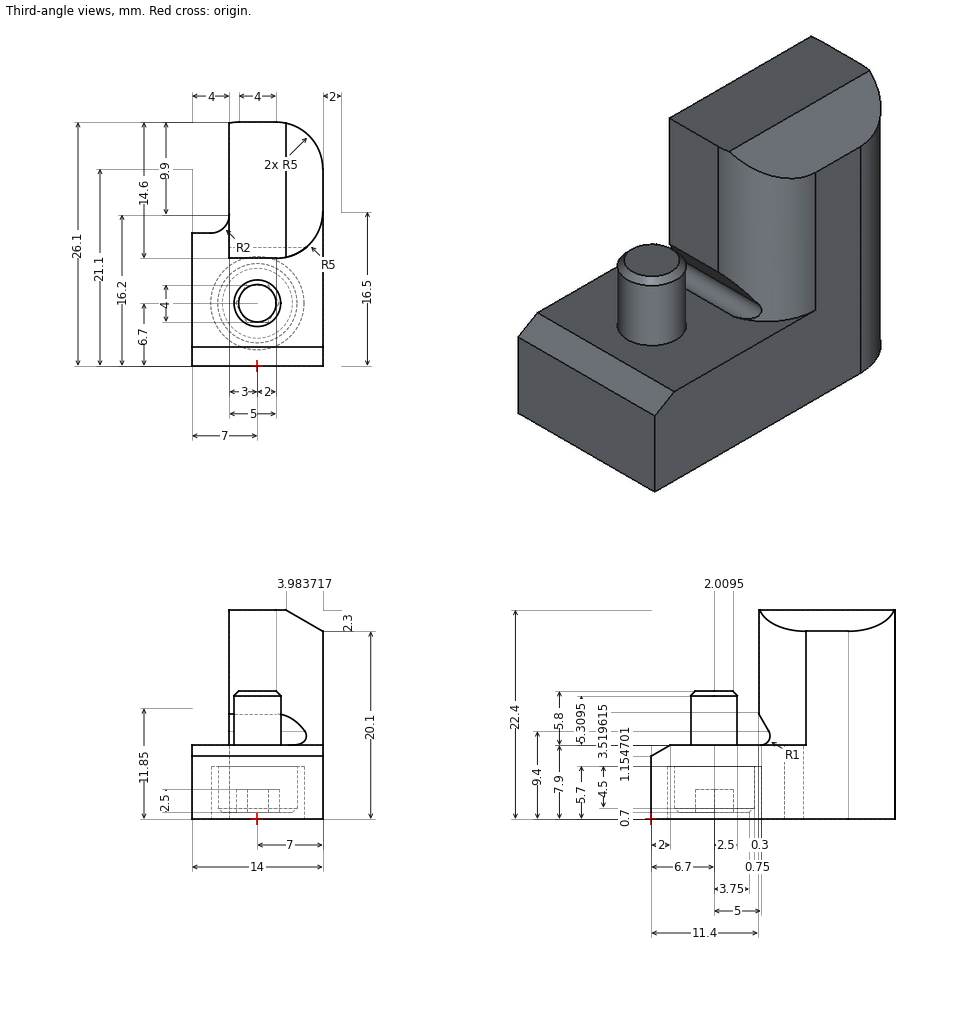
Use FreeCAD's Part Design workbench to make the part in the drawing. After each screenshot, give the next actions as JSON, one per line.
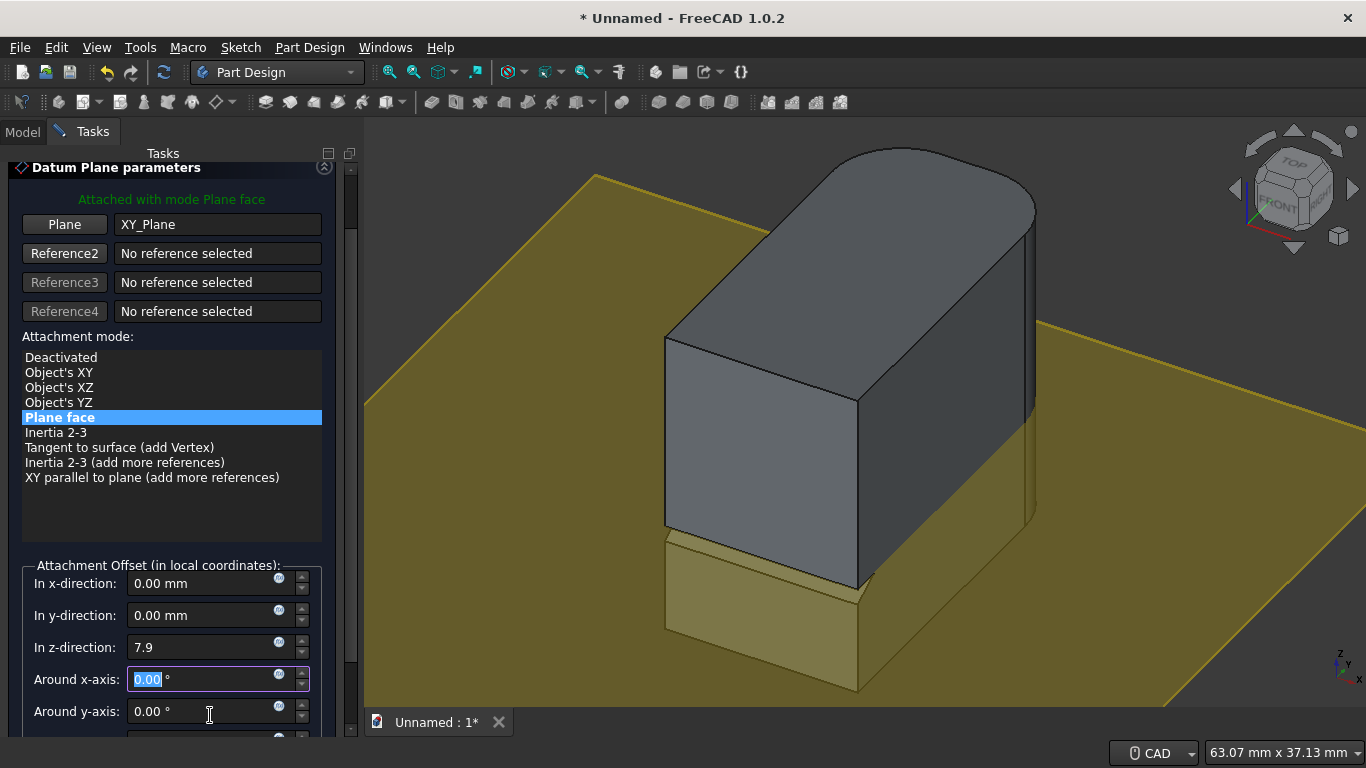
{"action": "scroll", "coordinate": [351, 450], "scroll_direction": "up", "scroll_amount": 2}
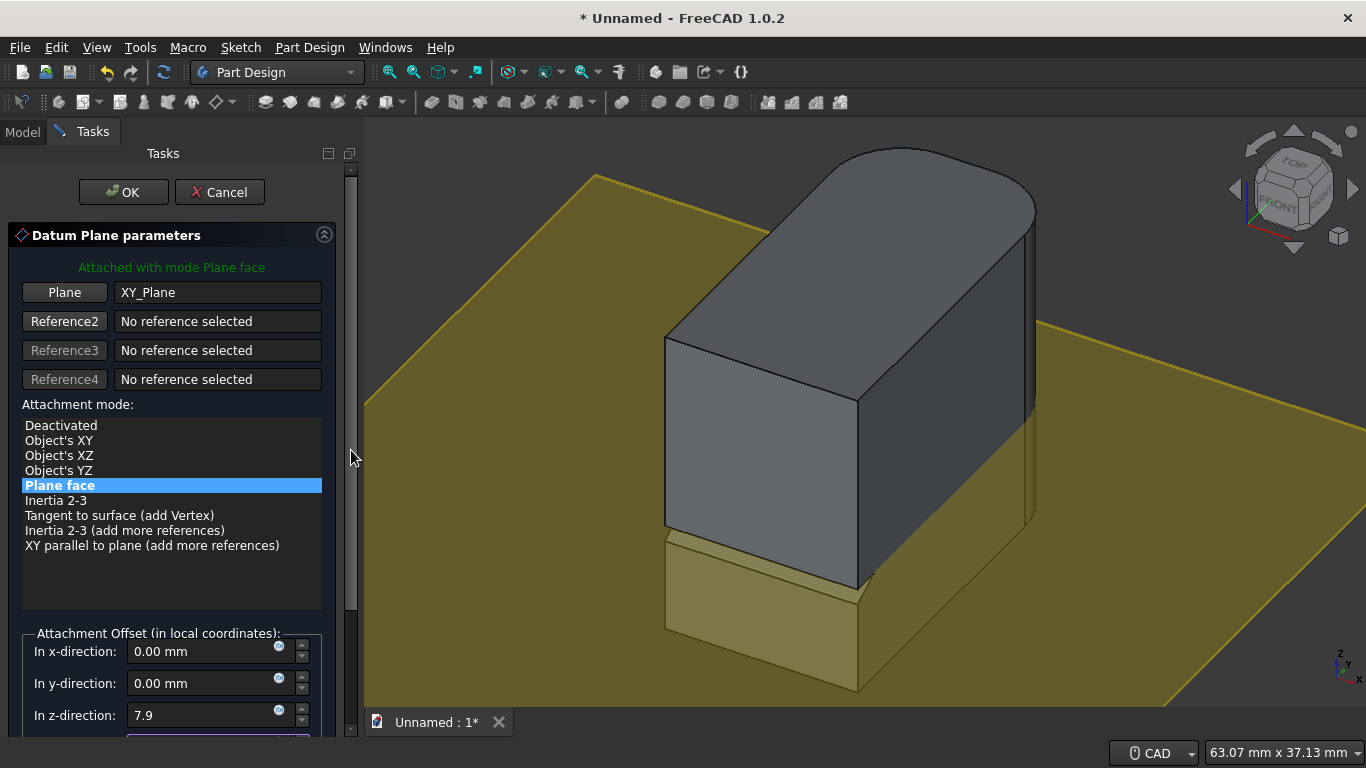
{"action": "left_click", "coordinate": [124, 192]}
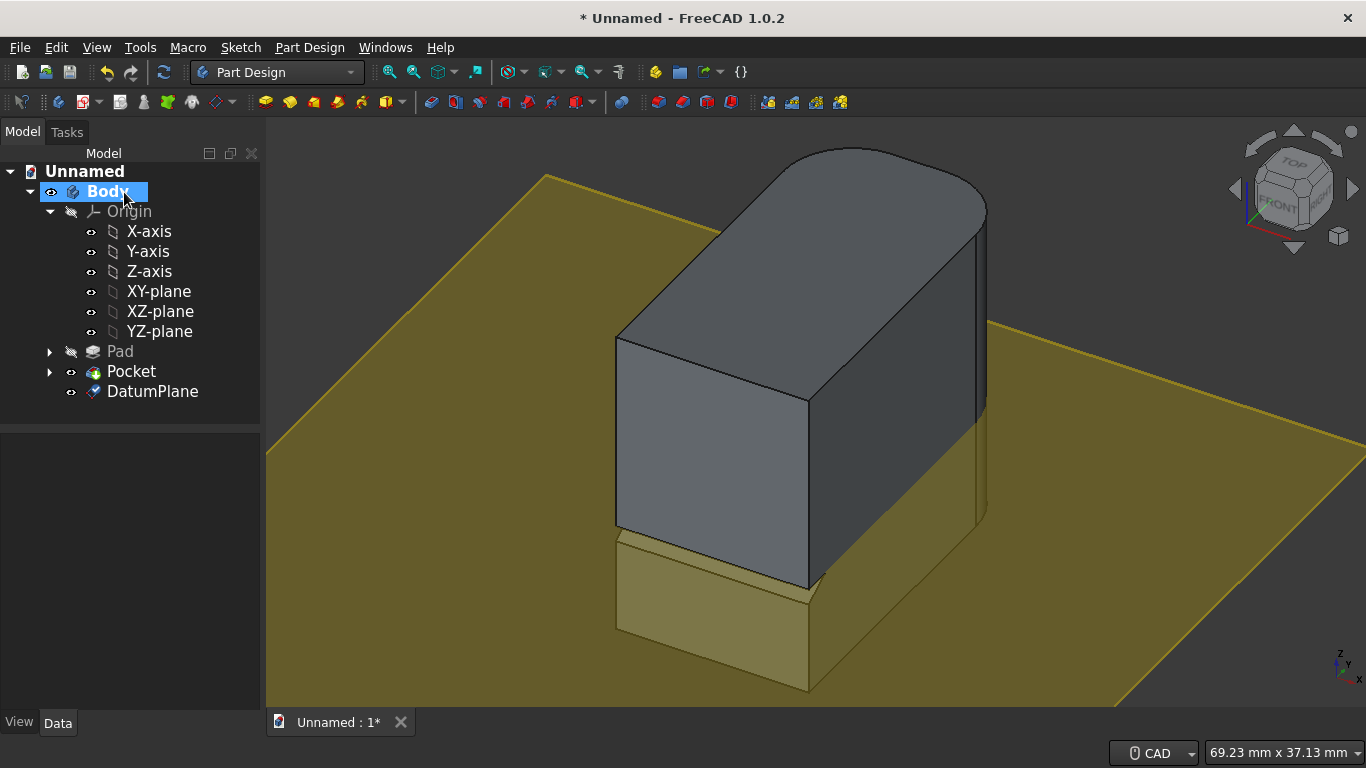
{"action": "left_click", "coordinate": [116, 392]}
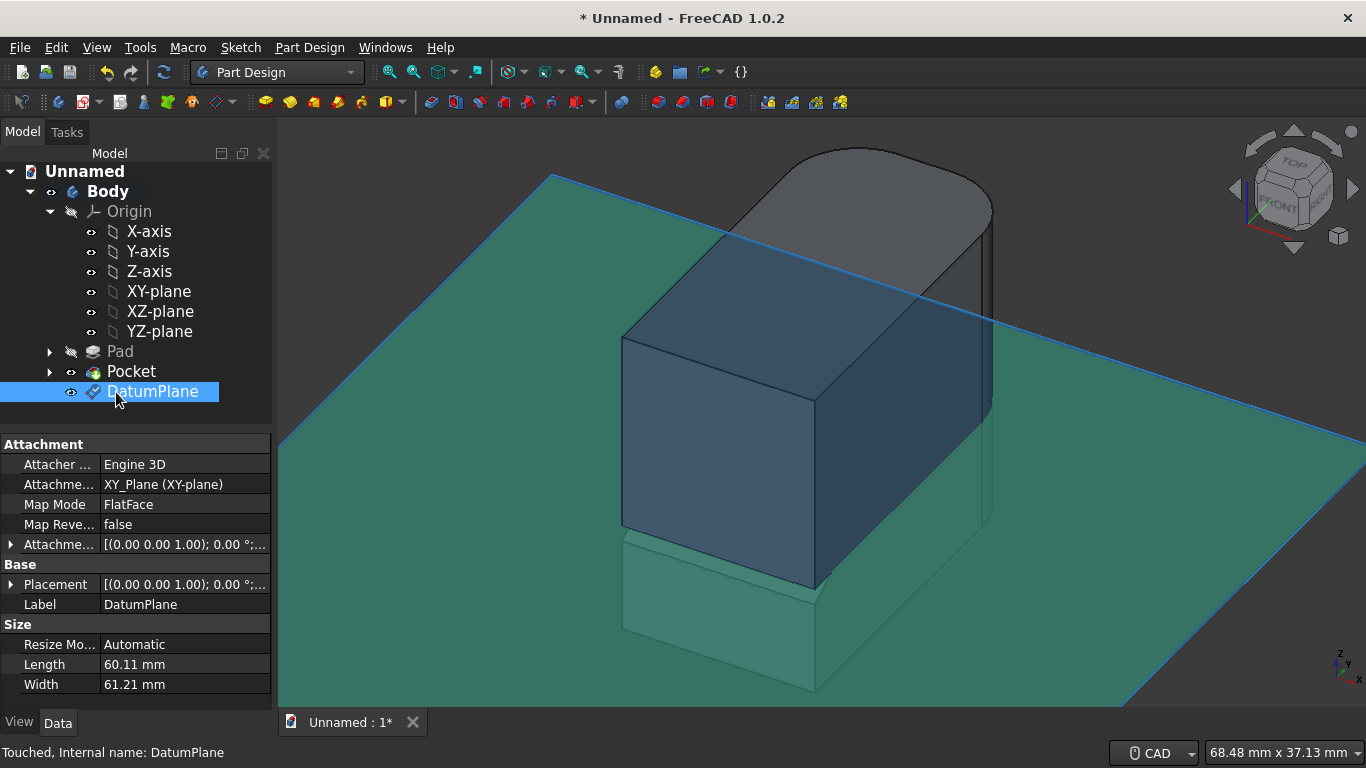
{"action": "left_click", "coordinate": [84, 102]}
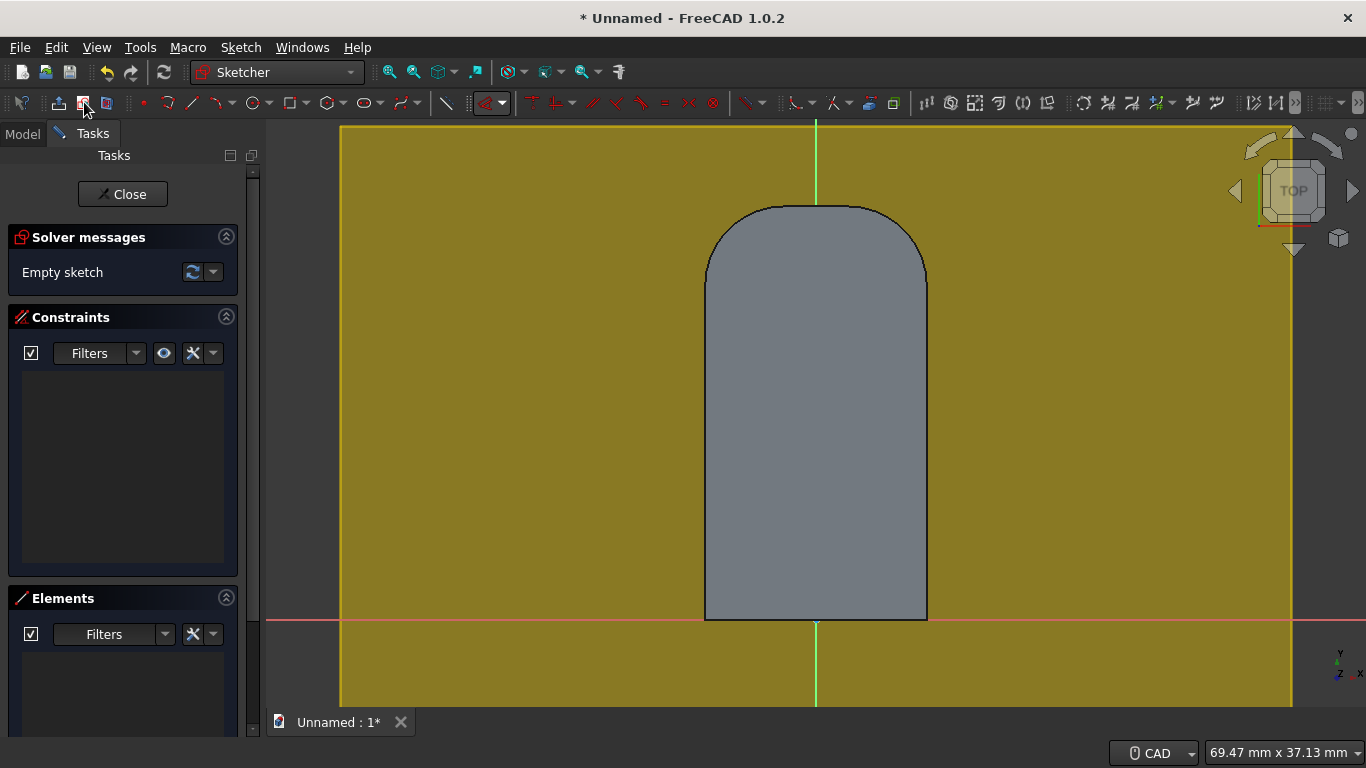
{"action": "left_click", "coordinate": [108, 104]}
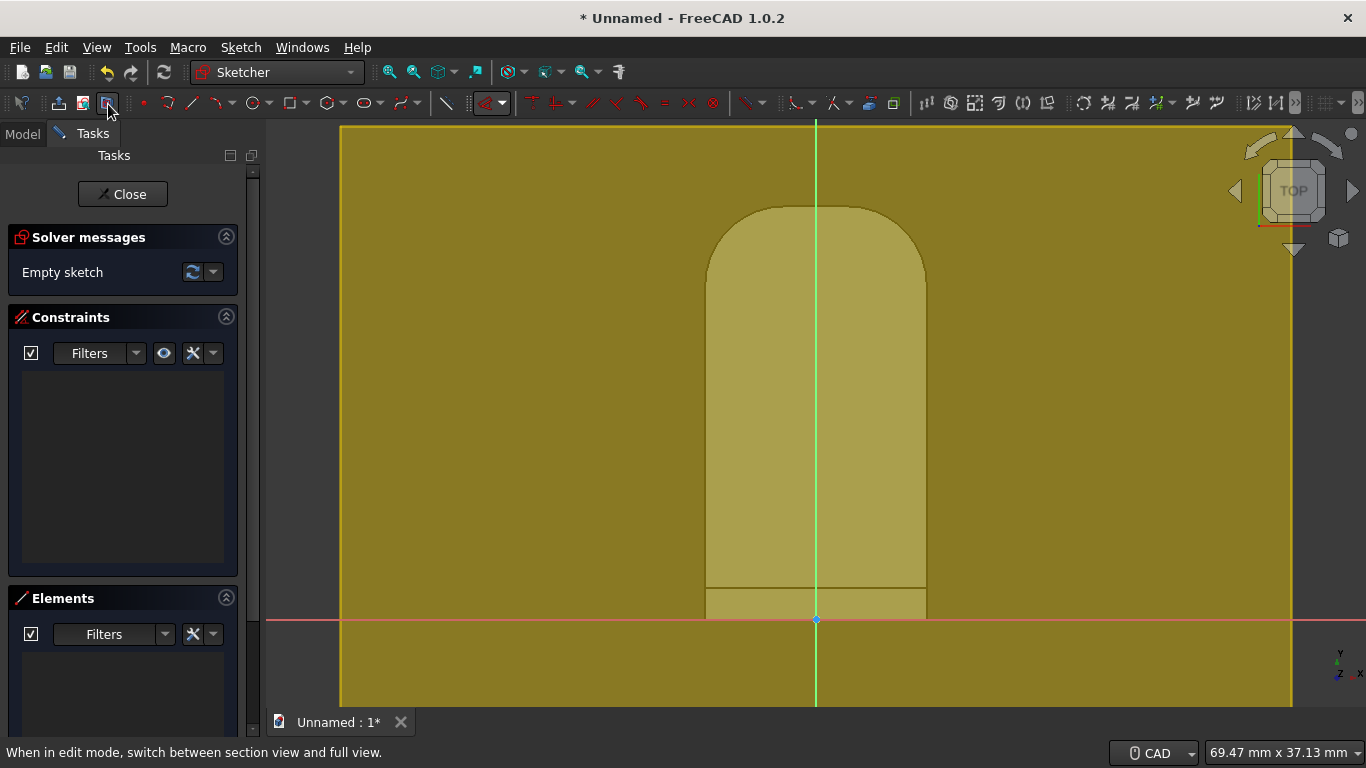
{"action": "left_click", "coordinate": [168, 104]}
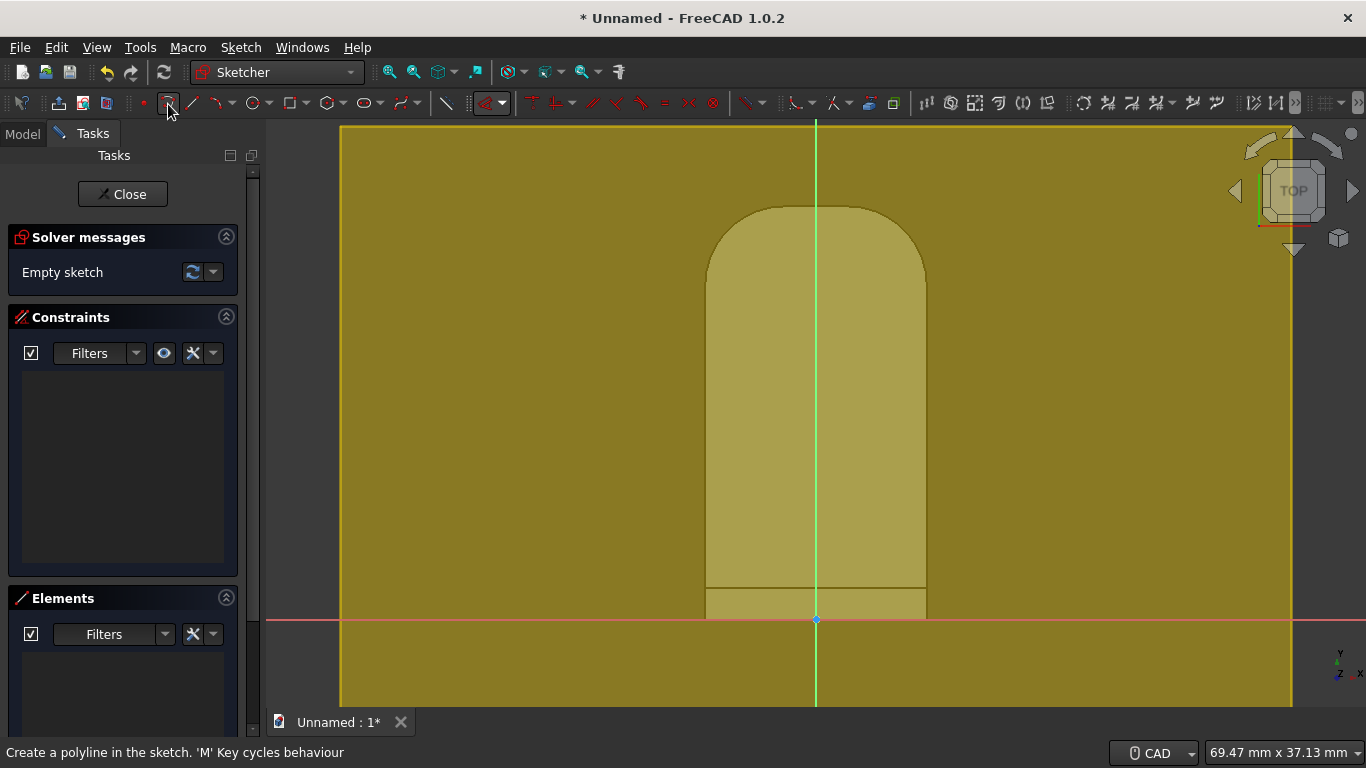
{"action": "left_click", "coordinate": [848, 438]}
{"action": "left_click", "coordinate": [768, 438]}
{"action": "left_click", "coordinate": [768, 206]}
{"action": "left_click", "coordinate": [705, 206]}
{"action": "left_click", "coordinate": [705, 620]}
{"action": "left_click", "coordinate": [959, 611]}
{"action": "left_click", "coordinate": [959, 358]}
{"action": "left_click", "coordinate": [927, 358]}
{"action": "right_click", "coordinate": [927, 358]}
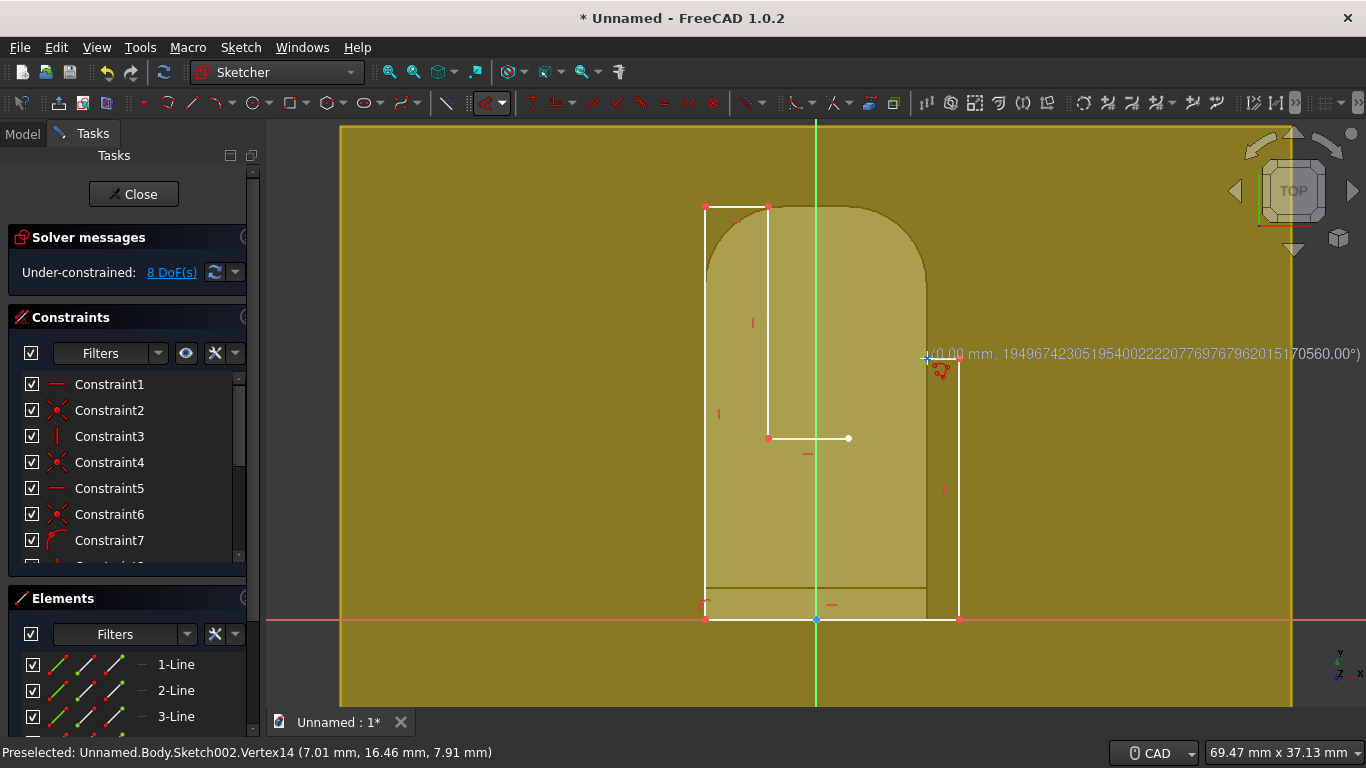
{"action": "left_click", "coordinate": [216, 104]}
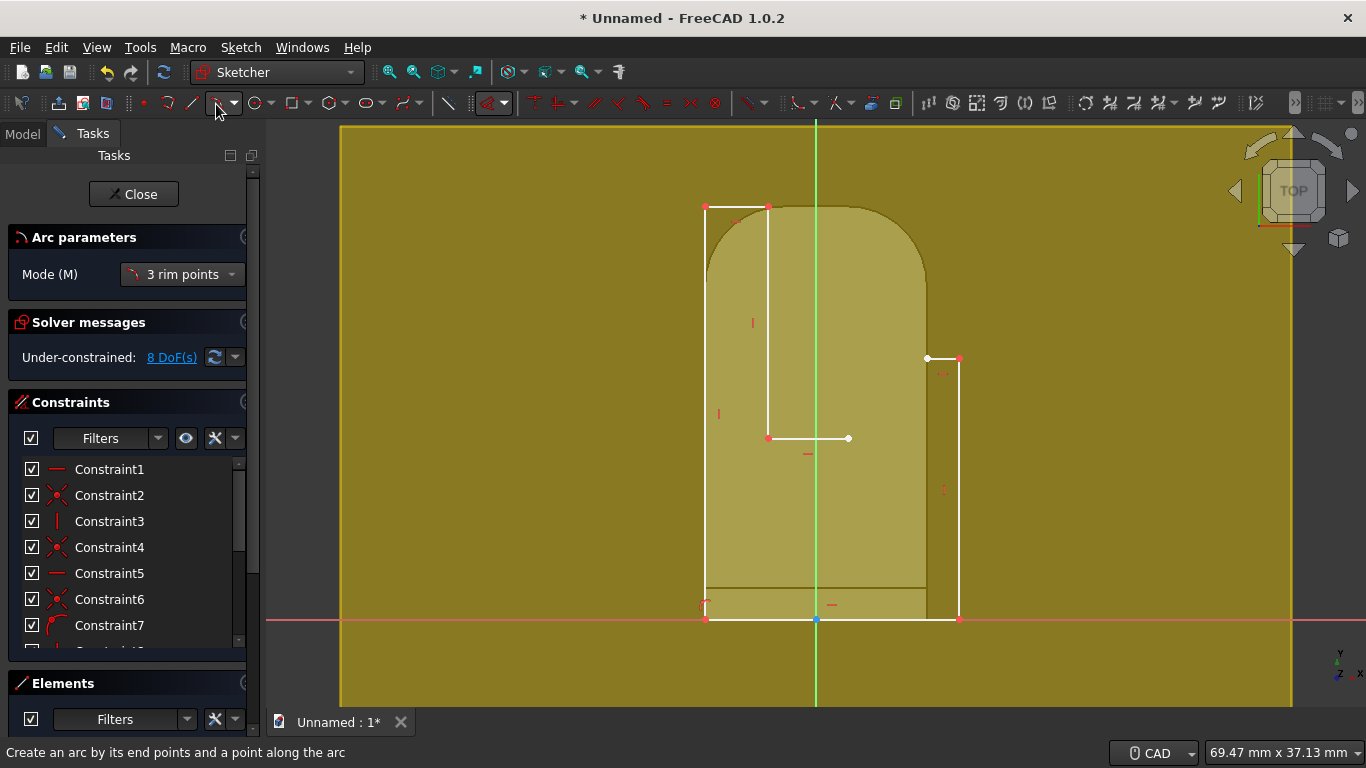
{"action": "left_click", "coordinate": [927, 359]}
{"action": "left_click", "coordinate": [848, 439]}
{"action": "left_click", "coordinate": [904, 414]}
{"action": "key", "text": "Escape"}